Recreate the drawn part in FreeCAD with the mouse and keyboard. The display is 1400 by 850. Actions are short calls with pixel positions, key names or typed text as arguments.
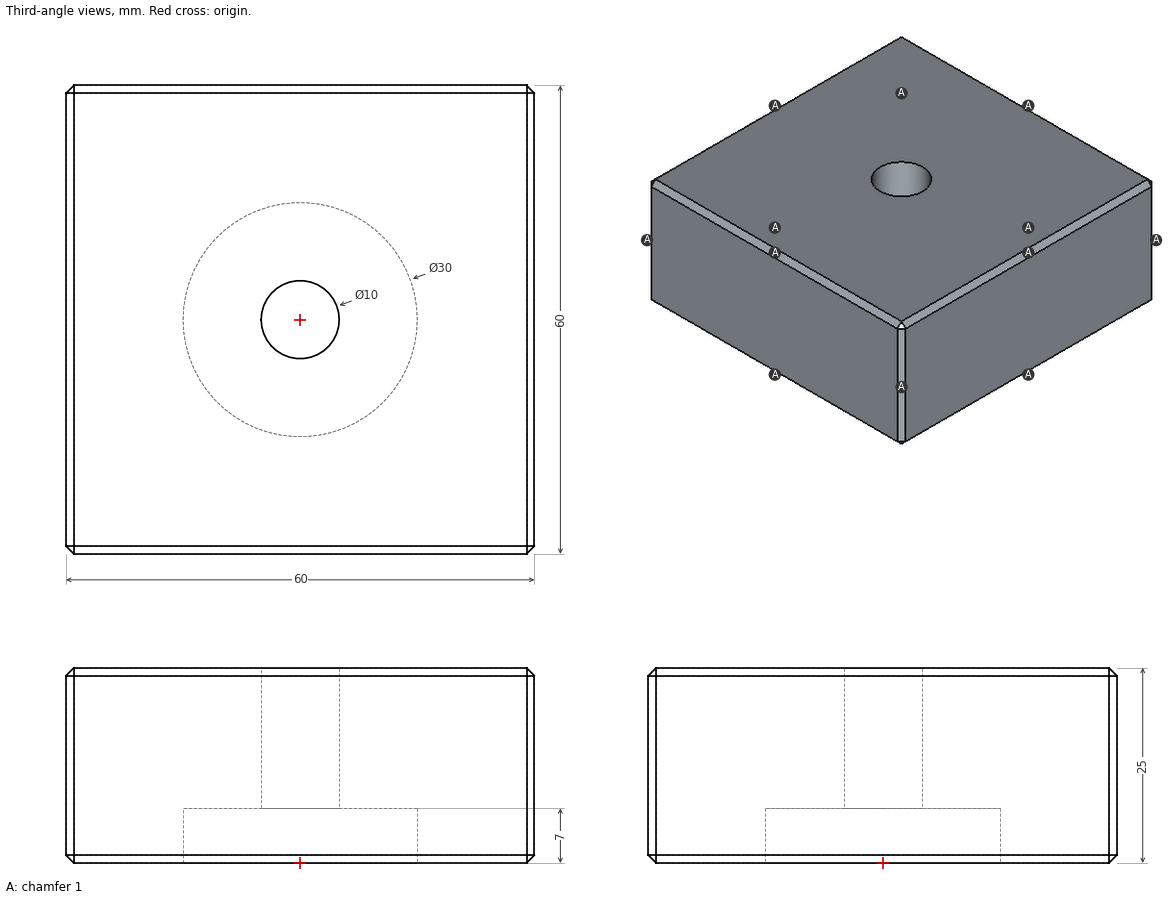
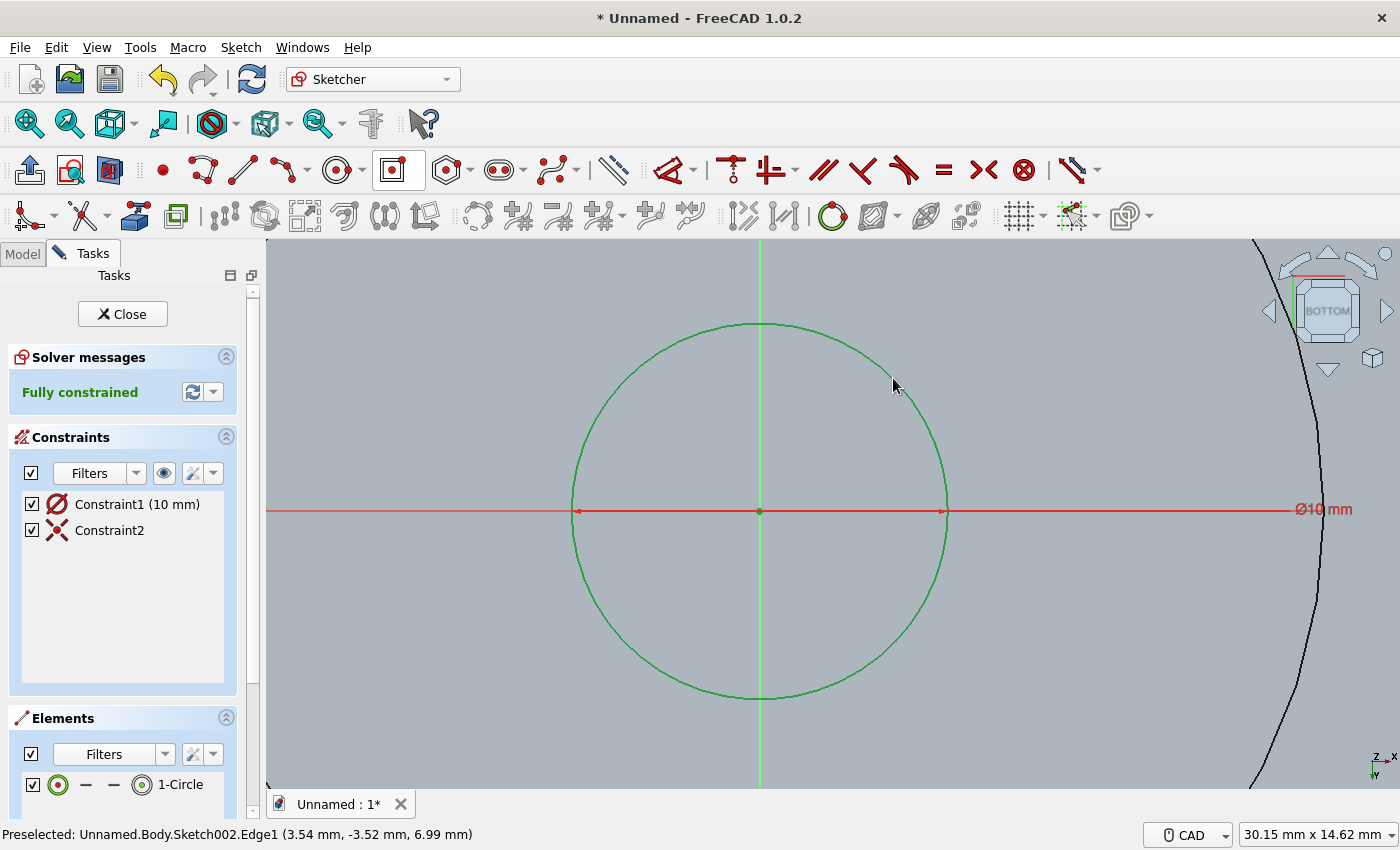
click(123, 314)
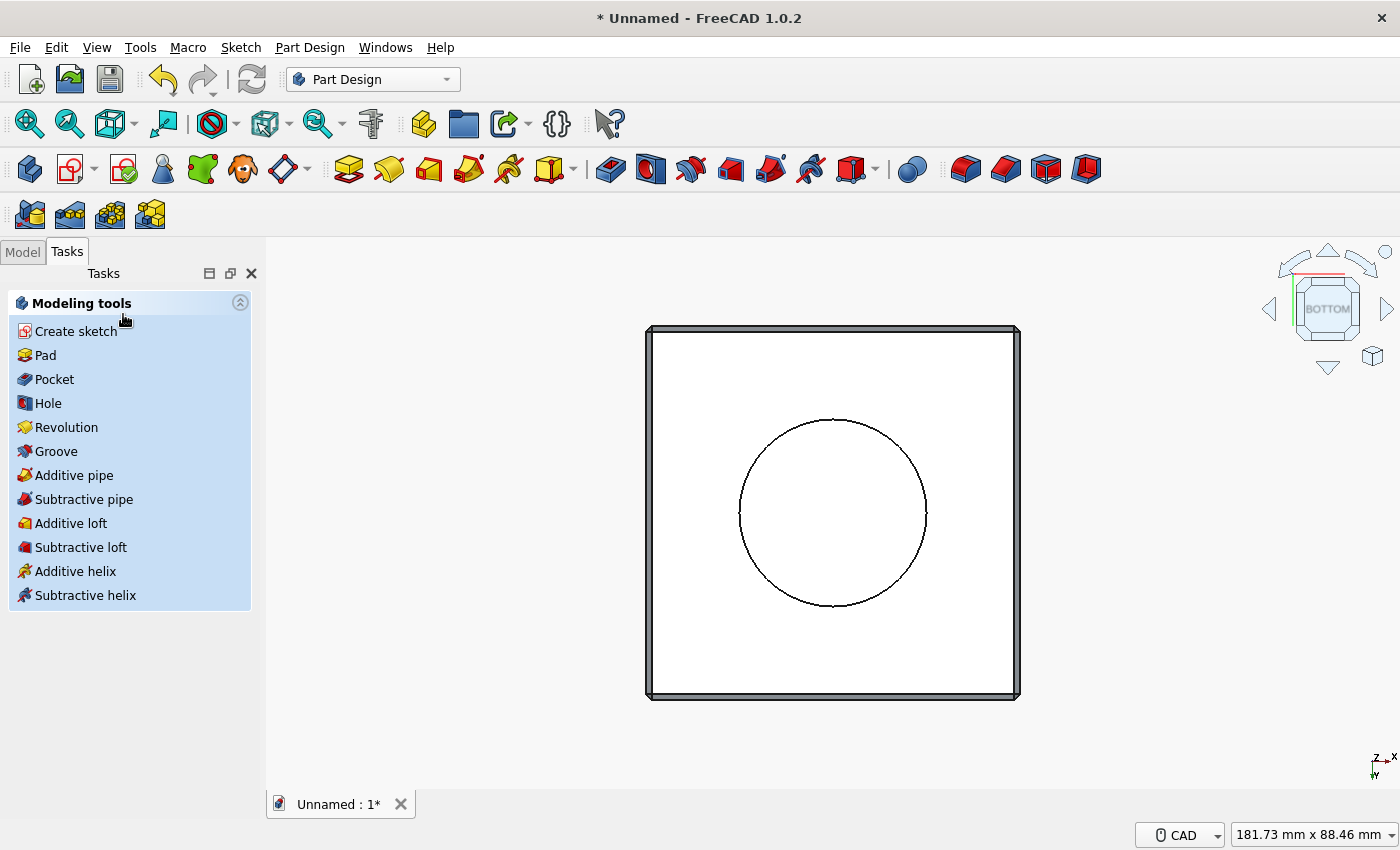
click(612, 170)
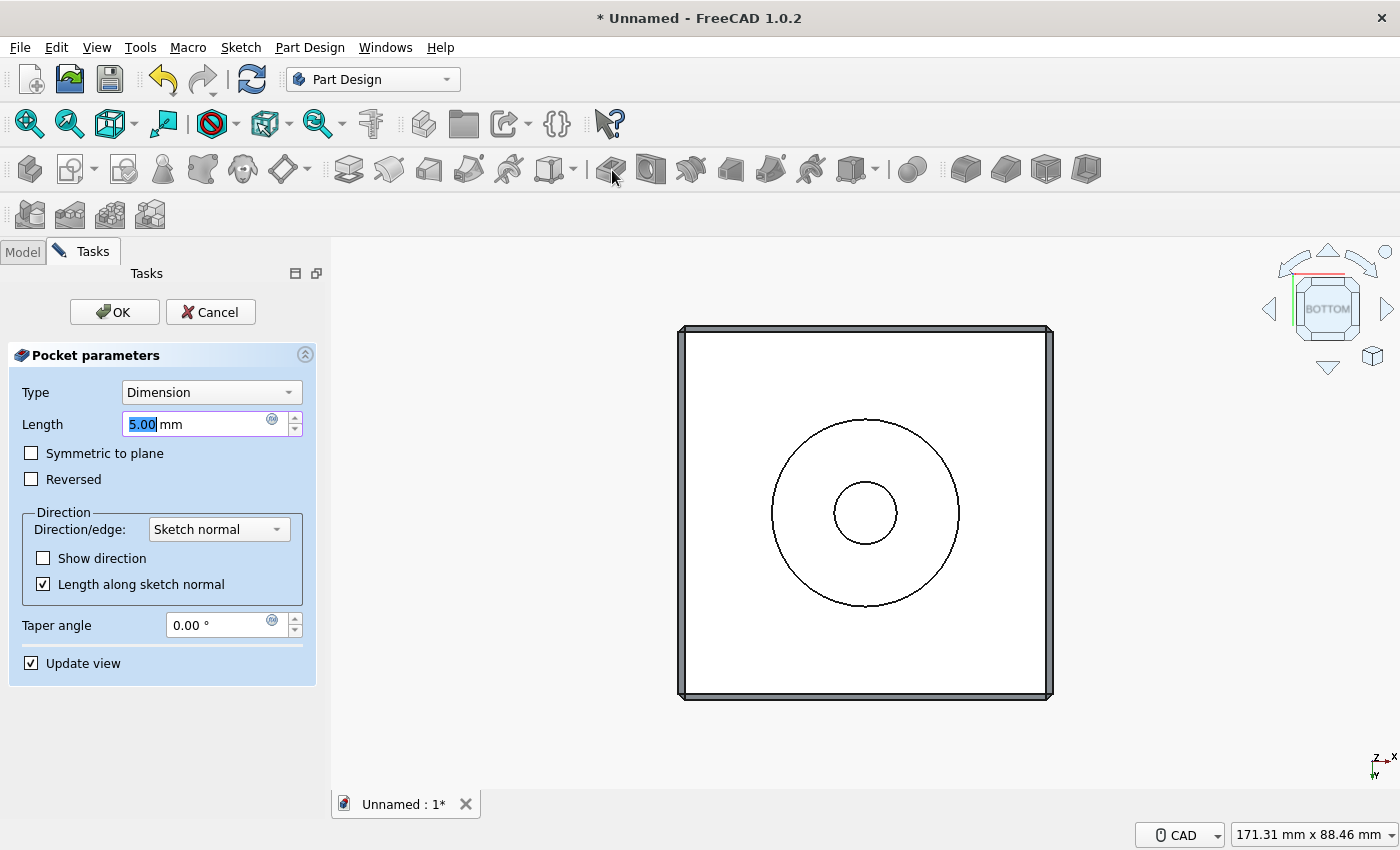
click(212, 392)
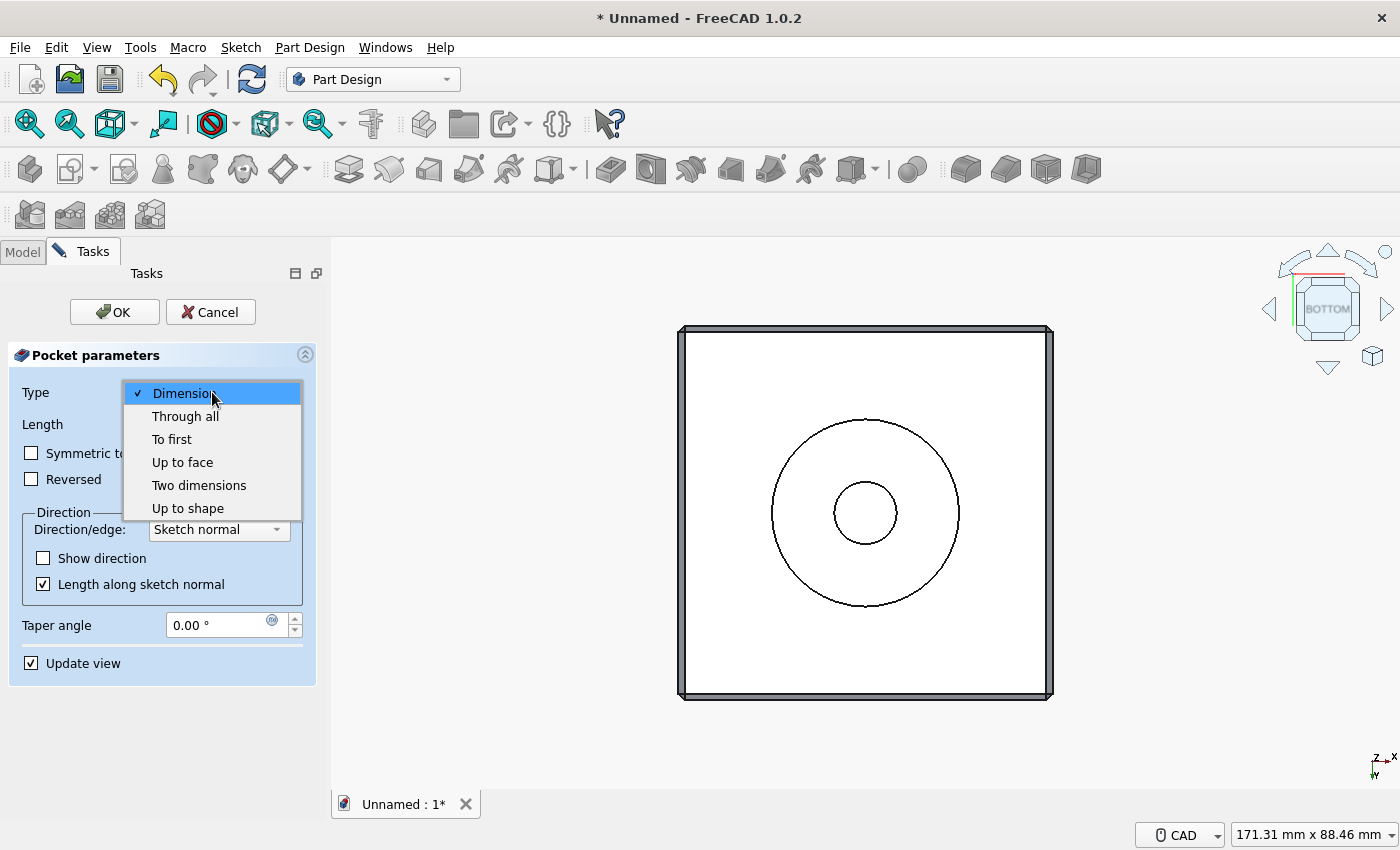
click(212, 416)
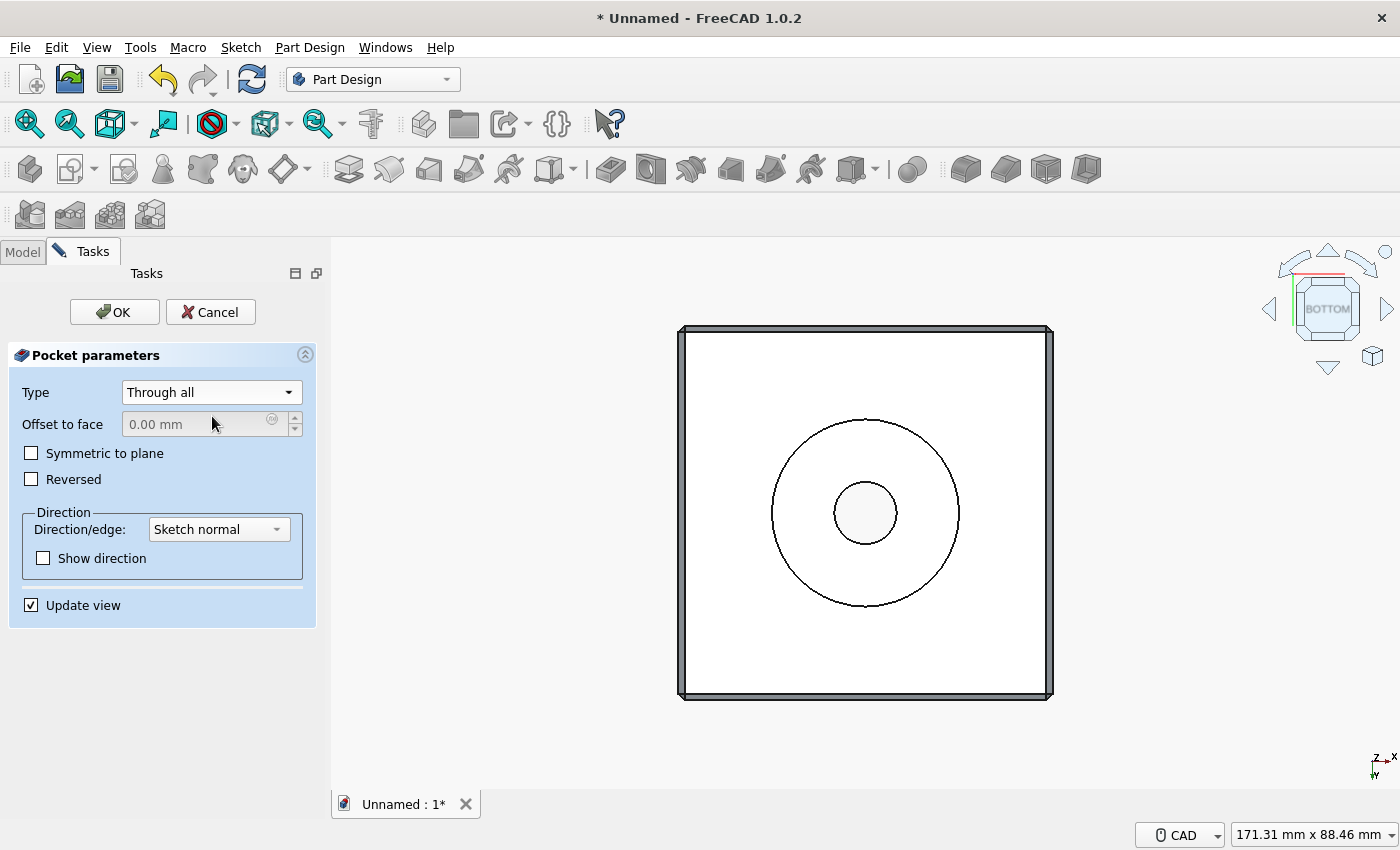
click(115, 312)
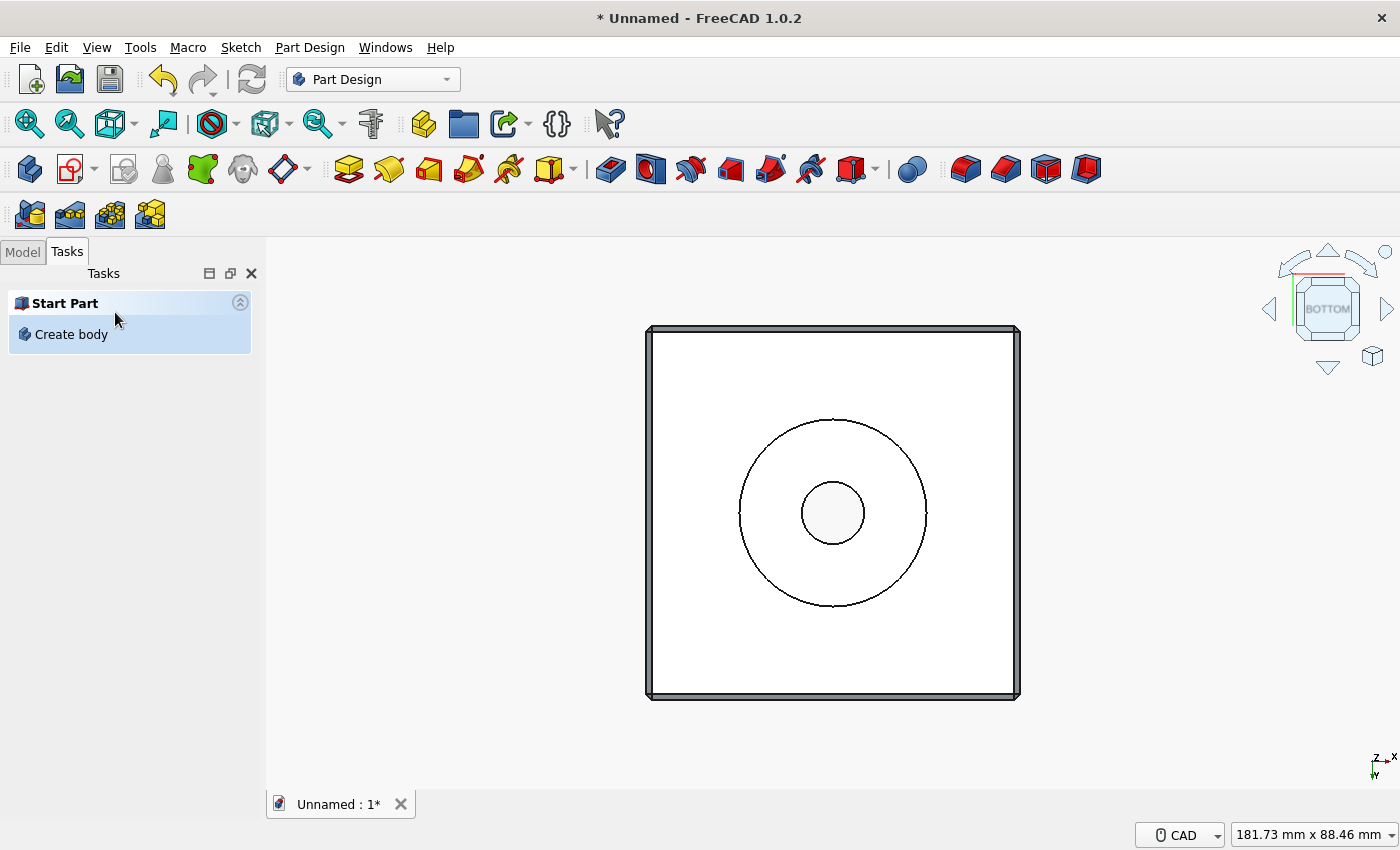
key(0)